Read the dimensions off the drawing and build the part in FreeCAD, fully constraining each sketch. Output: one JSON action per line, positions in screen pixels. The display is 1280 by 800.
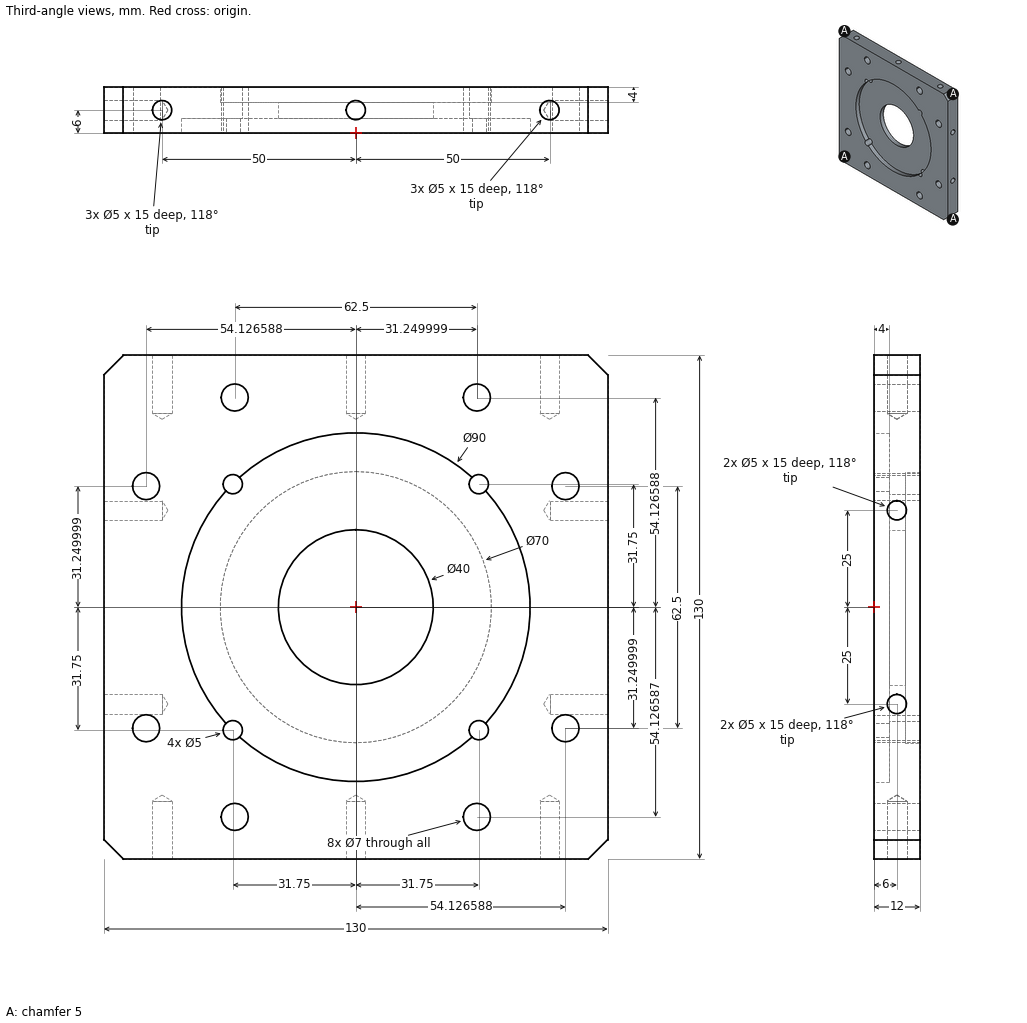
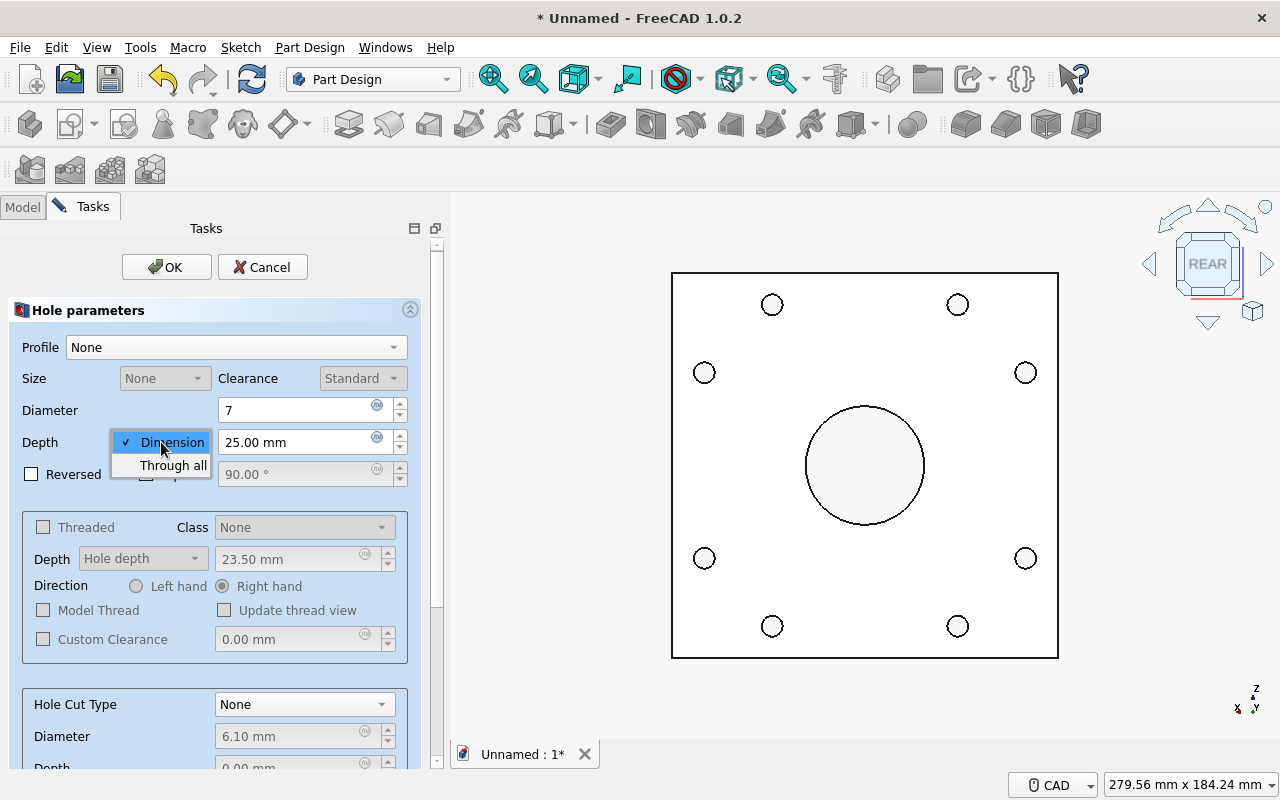
{"action": "left_click", "coordinate": [160, 466]}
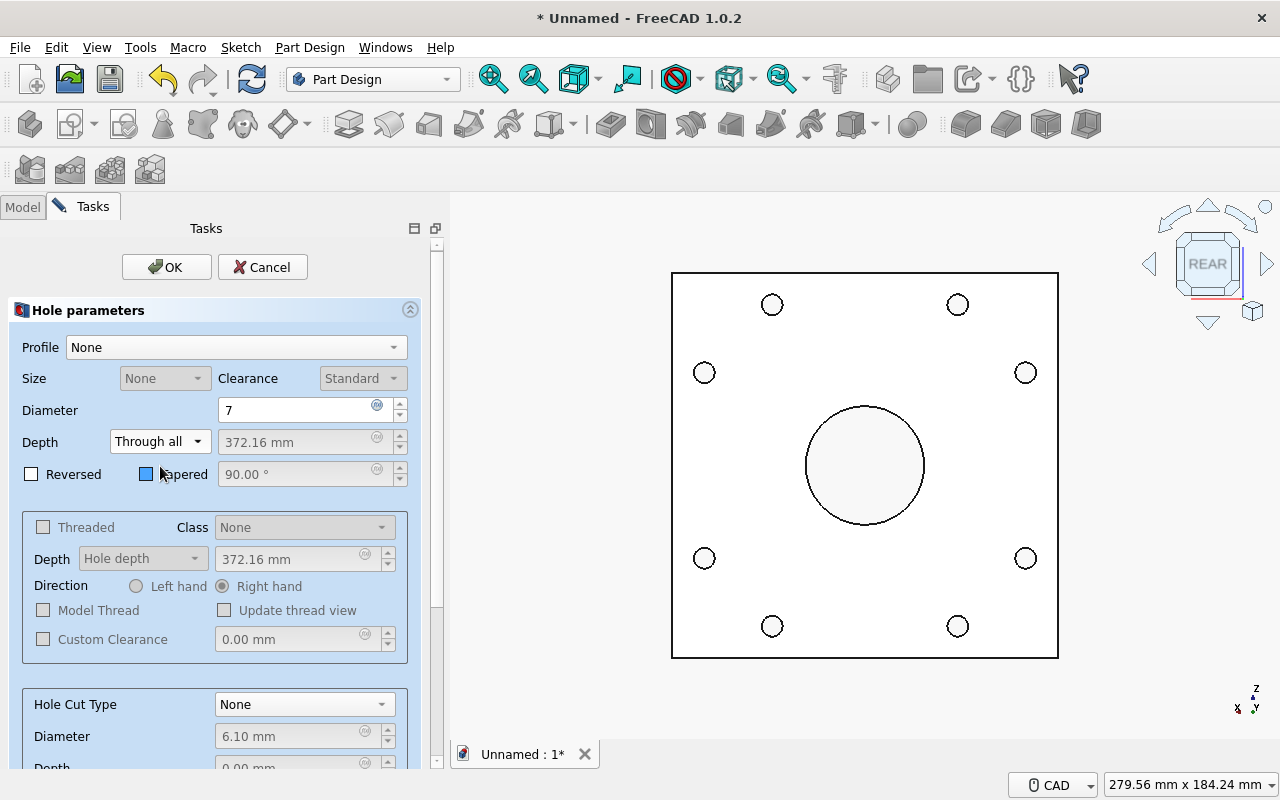
{"action": "left_click", "coordinate": [167, 267]}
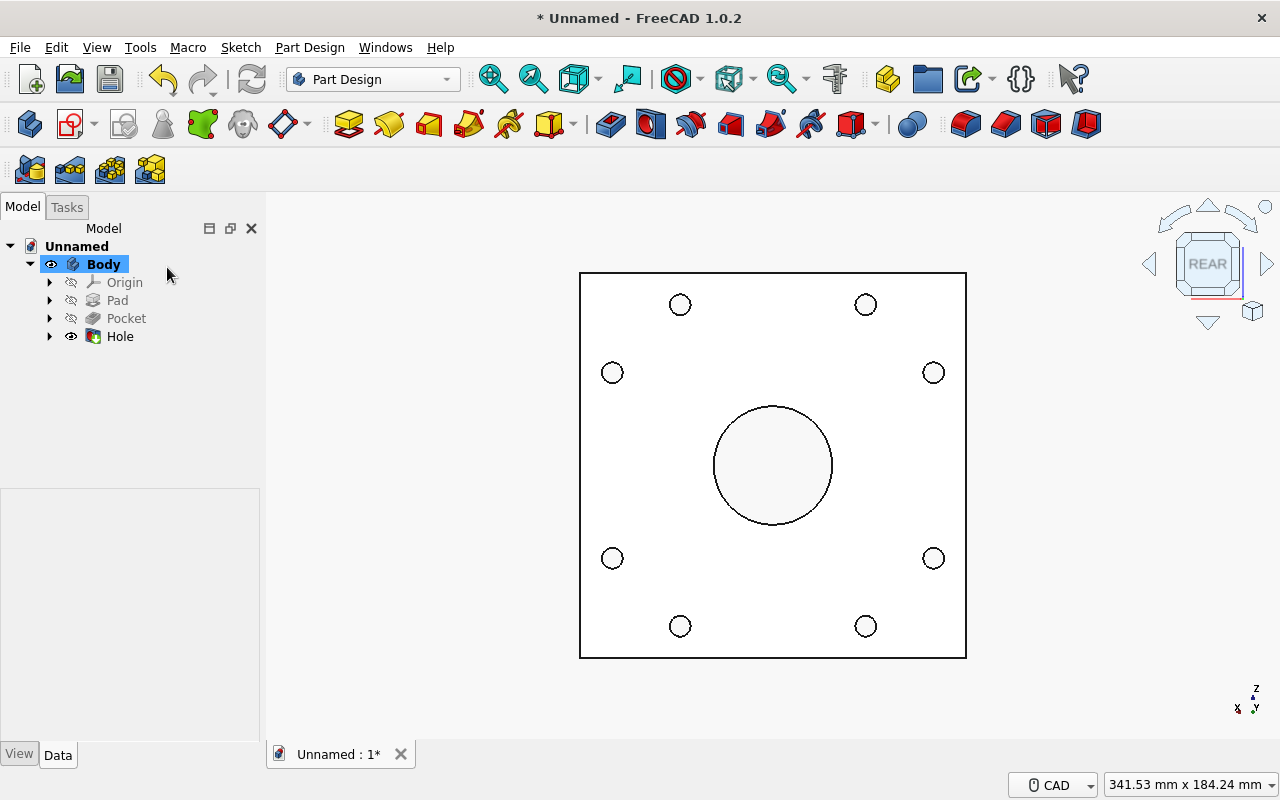
{"action": "left_click", "coordinate": [663, 409]}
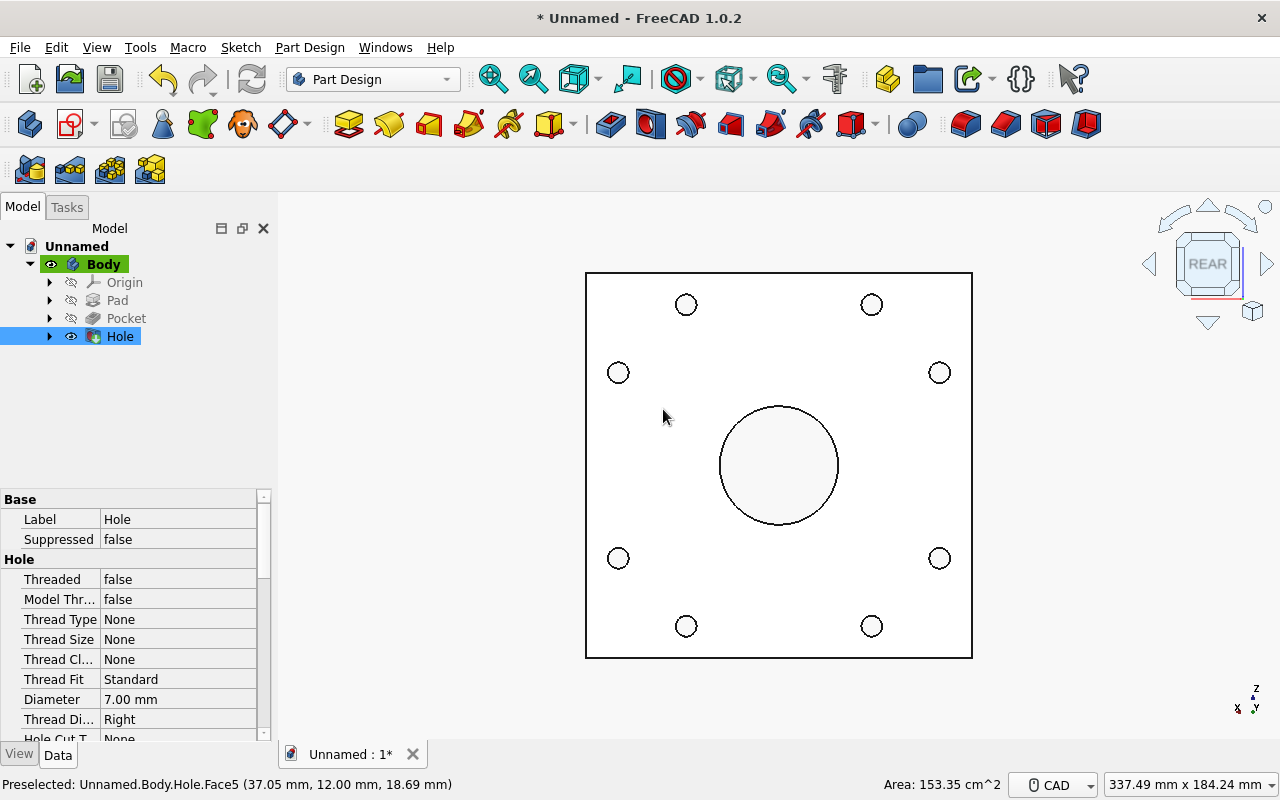
{"action": "left_click", "coordinate": [70, 124]}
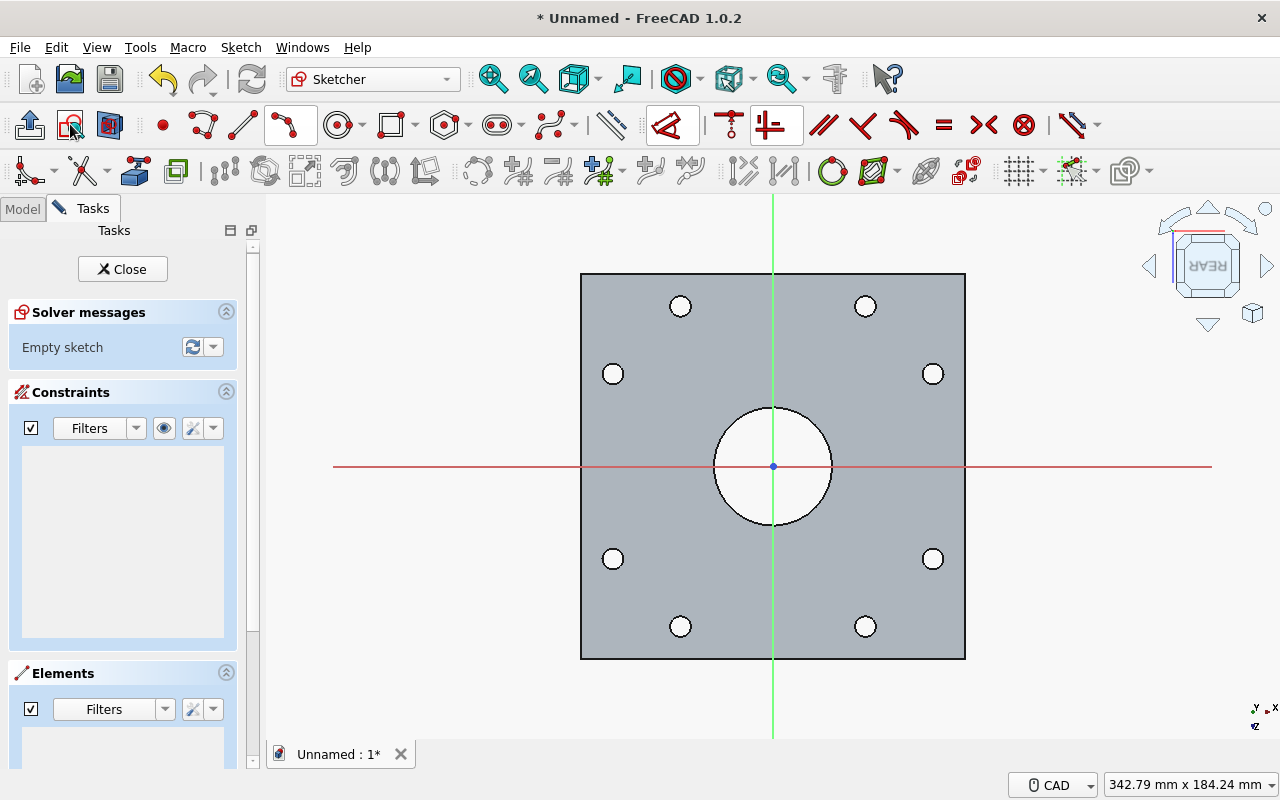
{"action": "scroll", "coordinate": [856, 466], "scroll_direction": "up", "scroll_amount": 3}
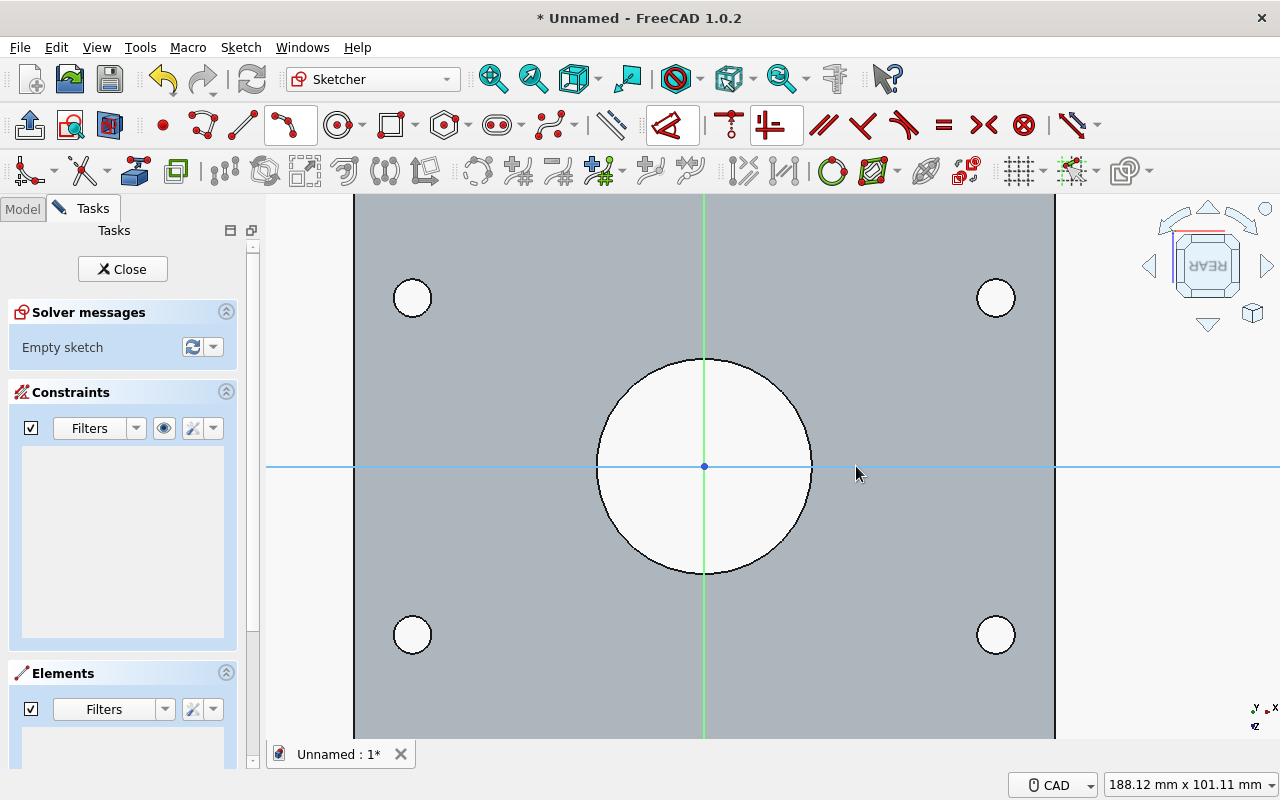
{"action": "key", "text": "g c"}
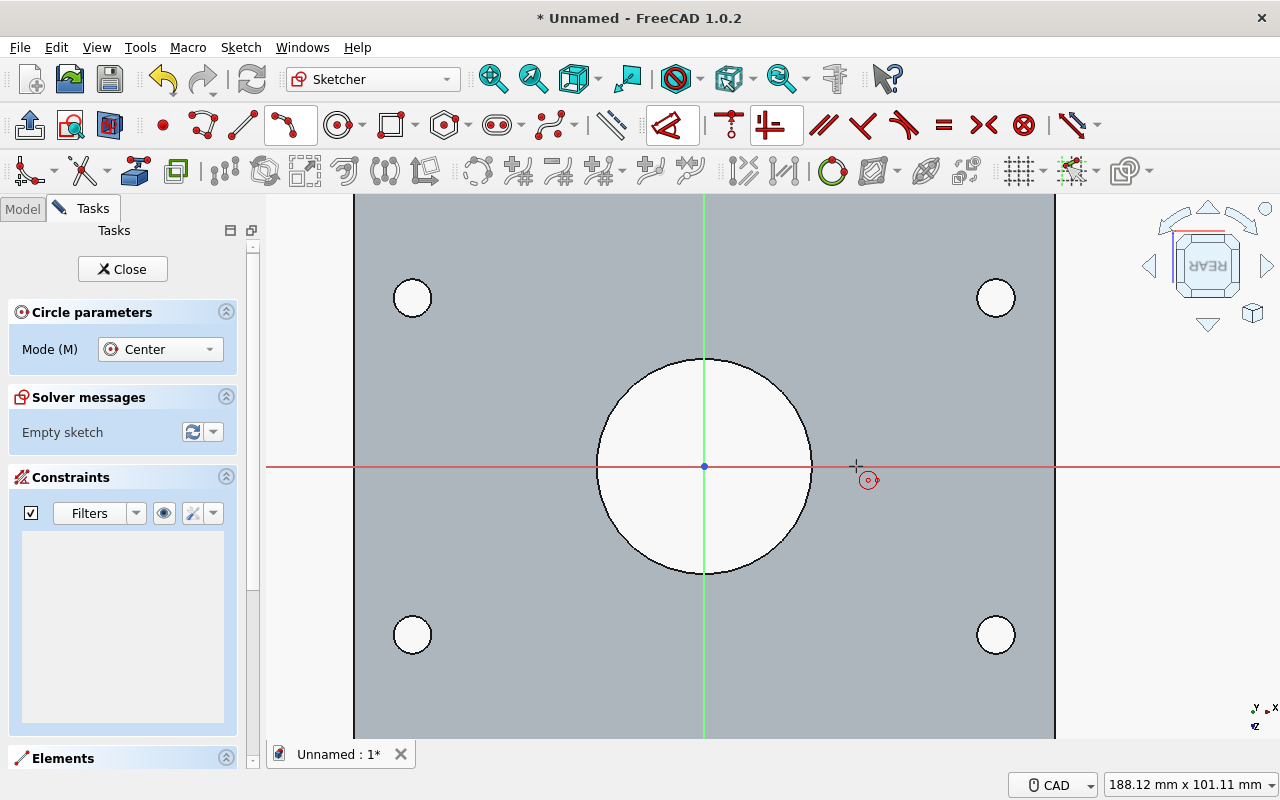
{"action": "left_click", "coordinate": [704, 466]}
{"action": "left_click", "coordinate": [838, 333]}
{"action": "key", "text": "Escape"}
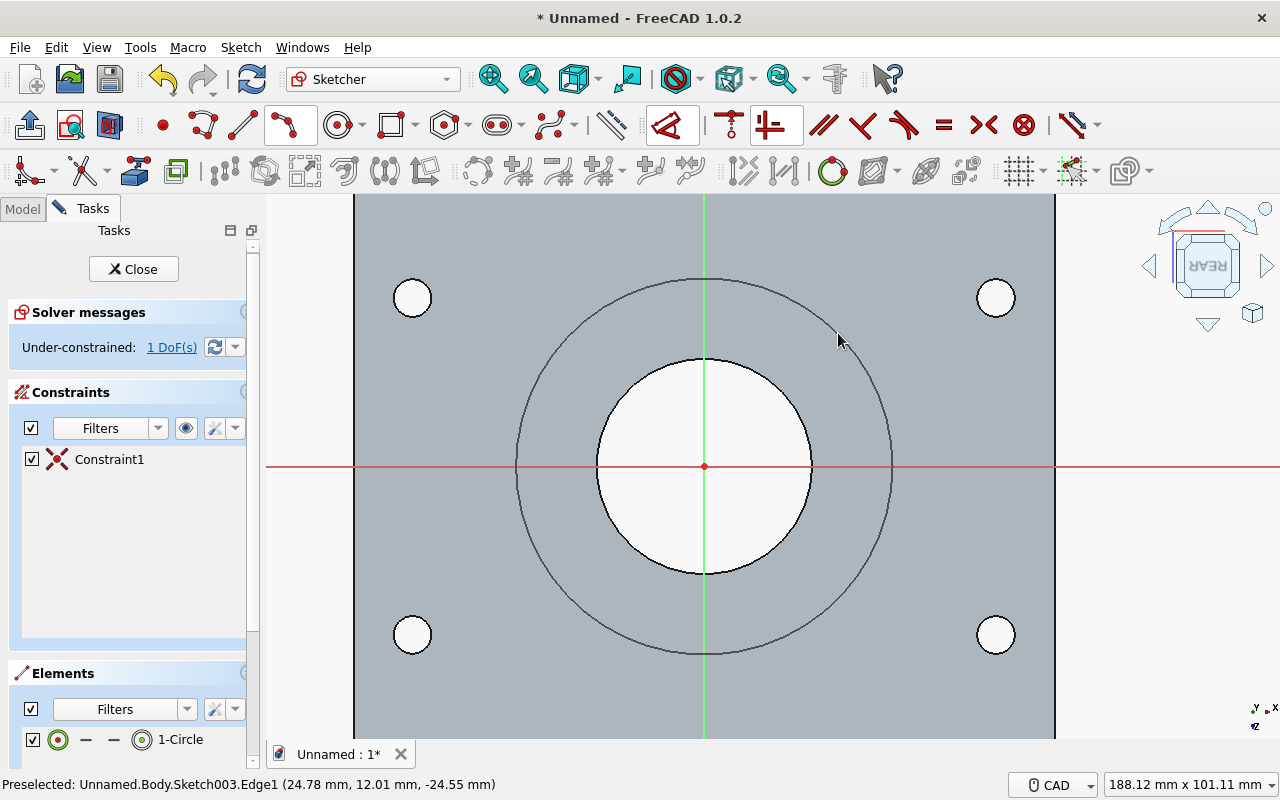
{"action": "key", "text": "d"}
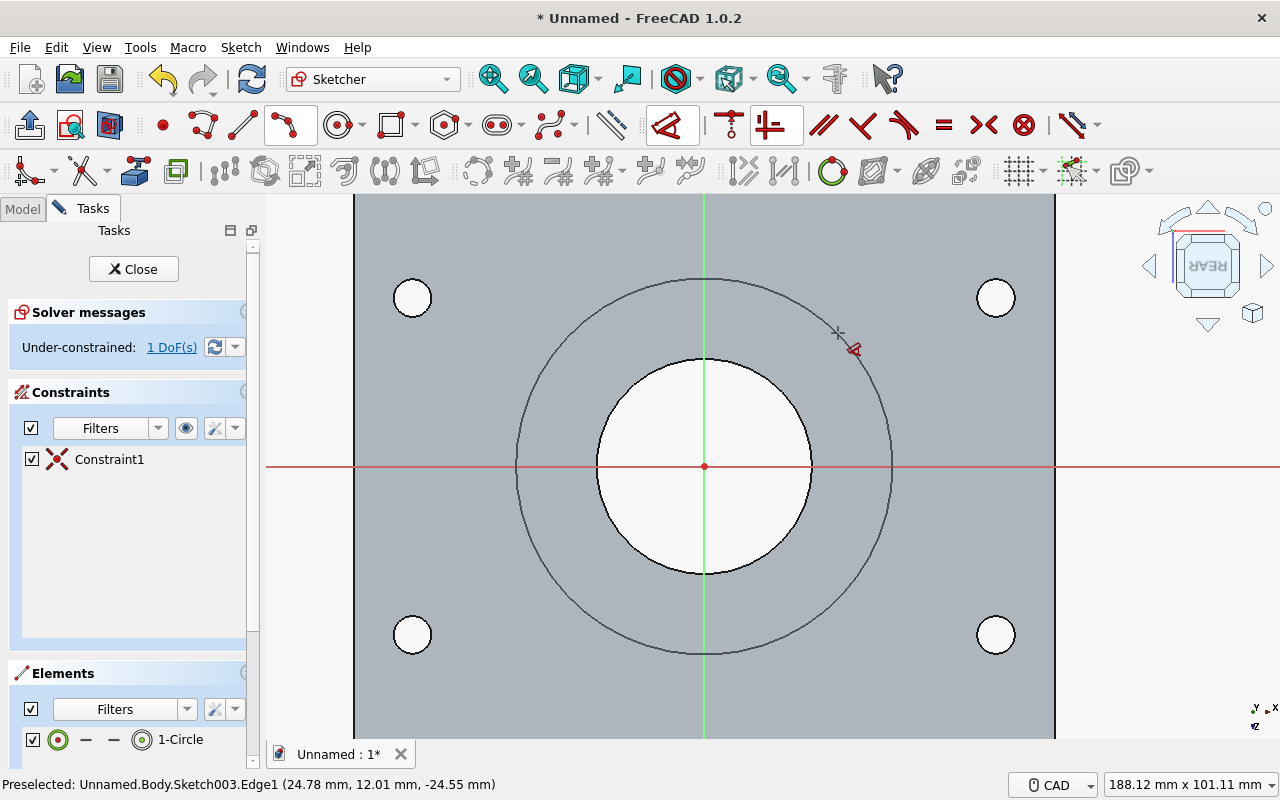
{"action": "left_click", "coordinate": [837, 333]}
{"action": "left_click", "coordinate": [860, 310]}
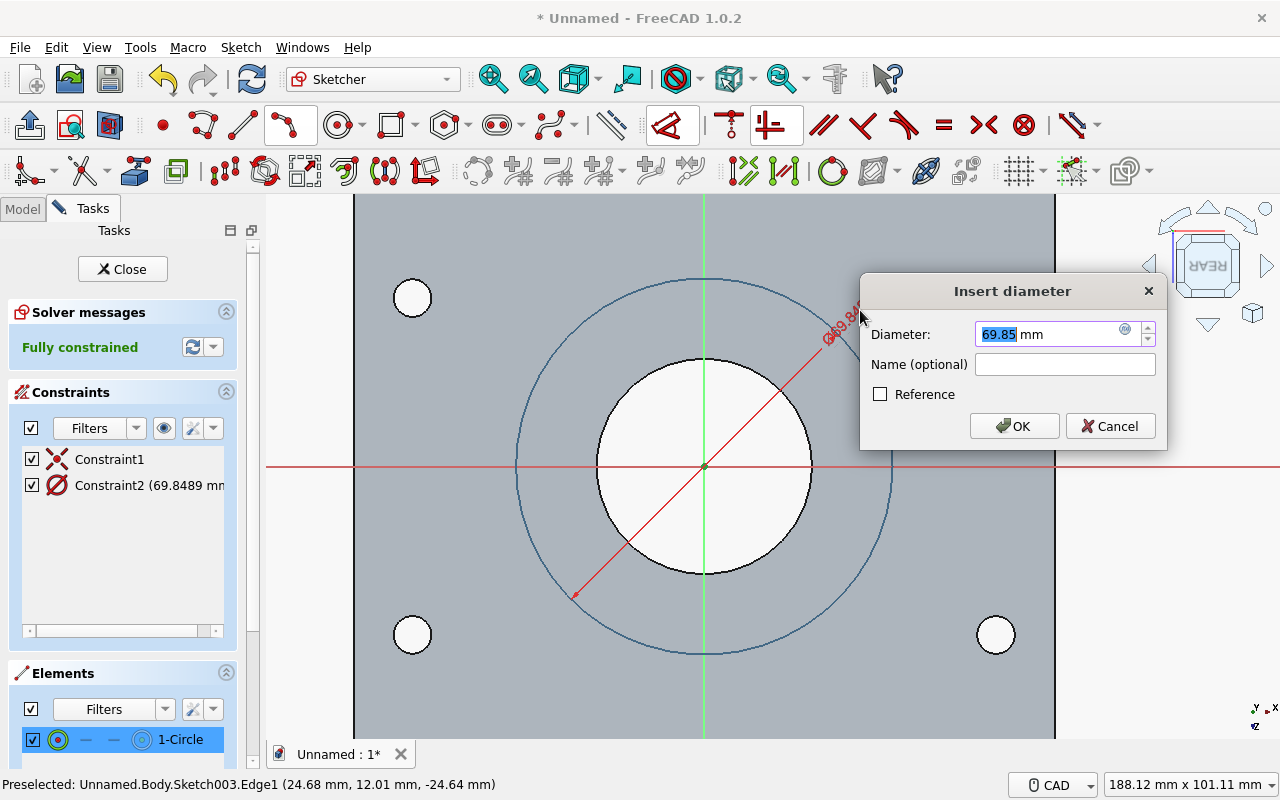
{"action": "type", "text": "70"}
{"action": "key", "text": "Return"}
{"action": "key", "text": "Escape"}